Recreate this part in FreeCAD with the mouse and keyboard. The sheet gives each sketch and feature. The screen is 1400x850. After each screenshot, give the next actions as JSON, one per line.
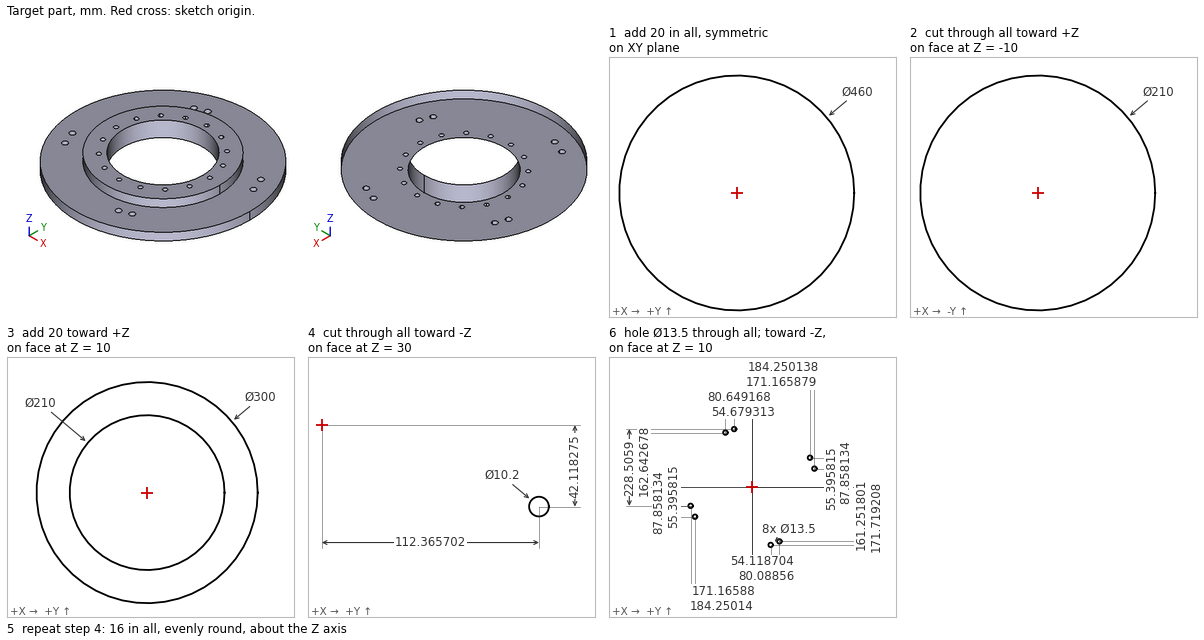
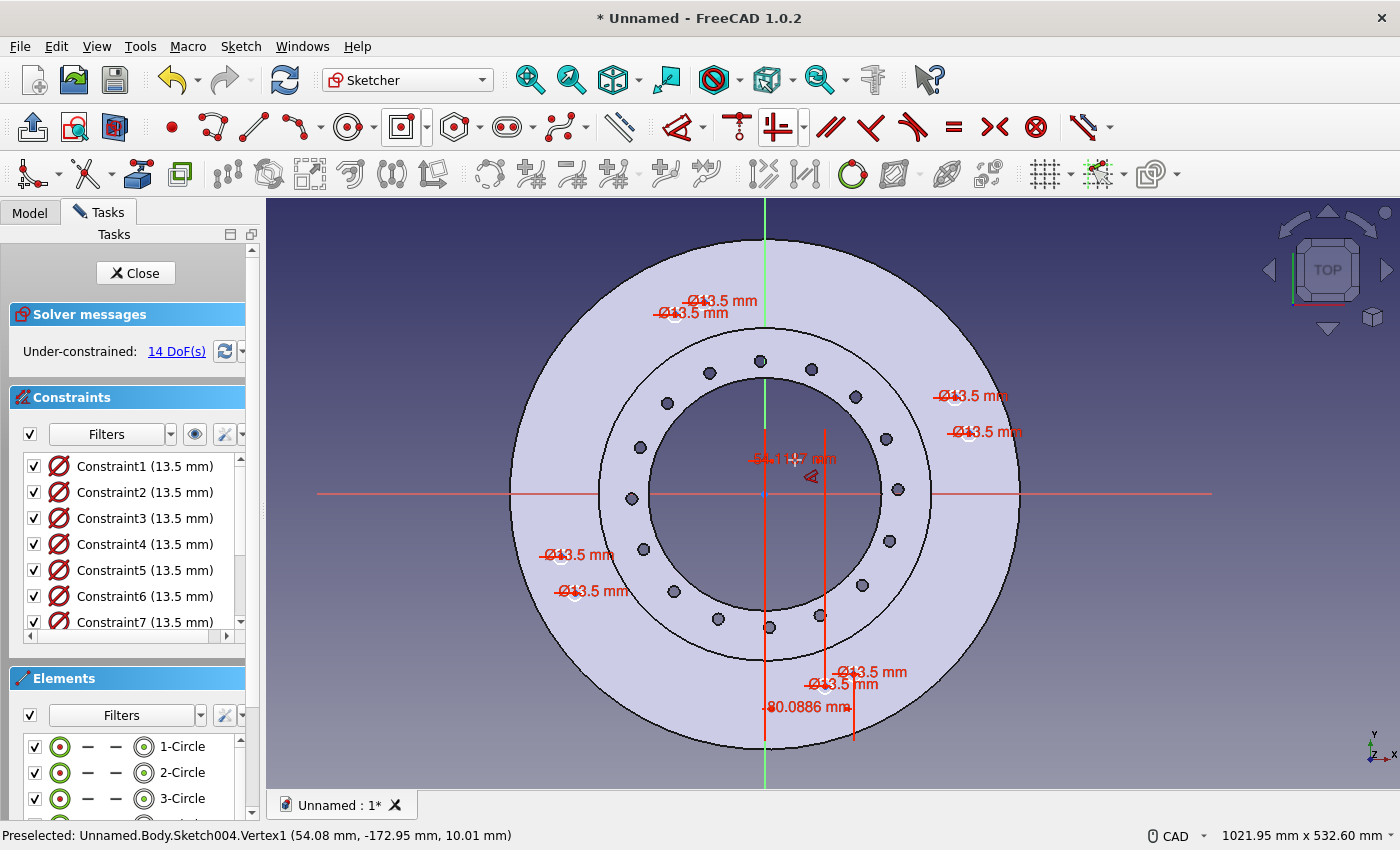
{"action": "left_click", "coordinate": [955, 398]}
{"action": "left_click", "coordinate": [989, 446]}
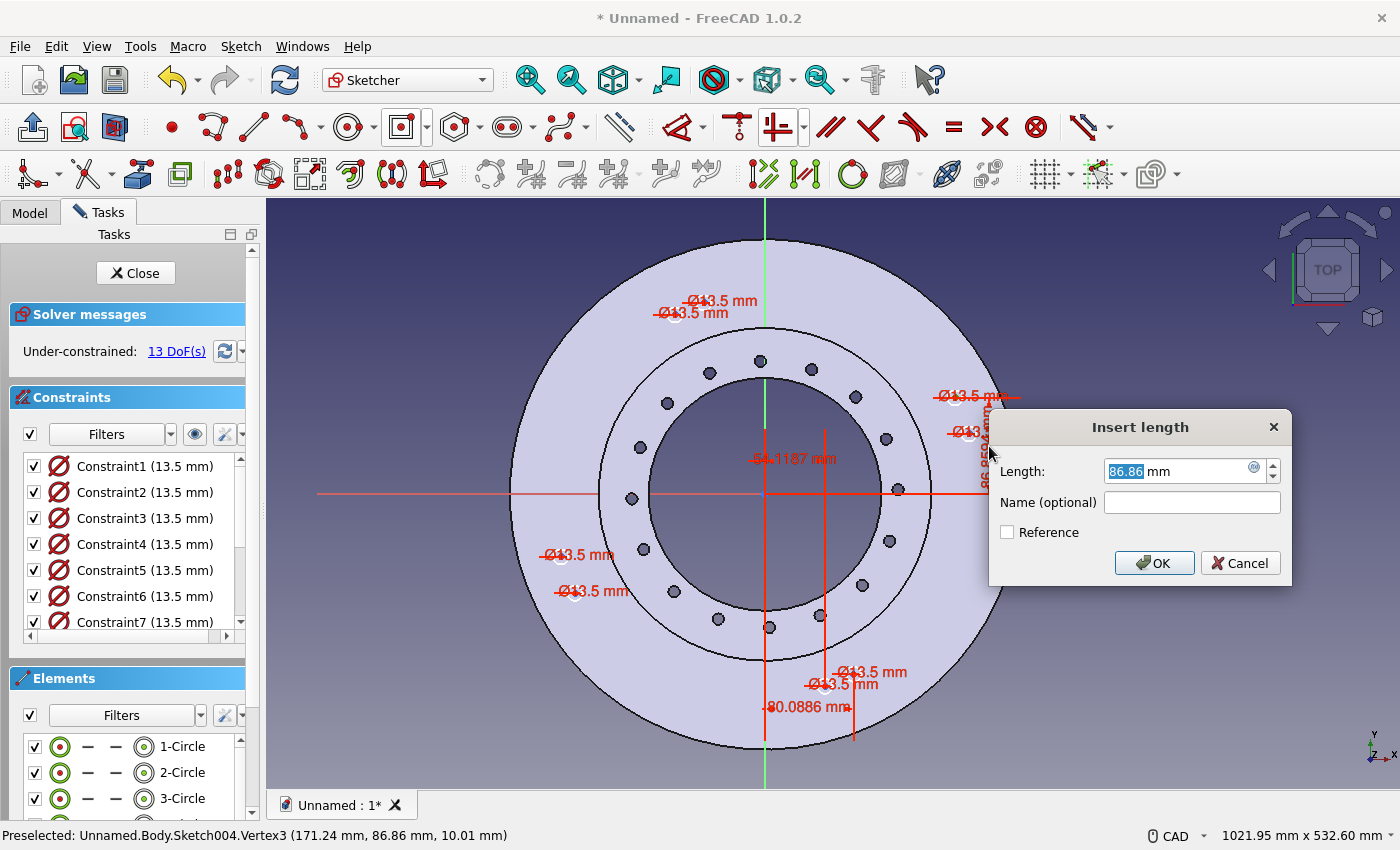
{"action": "type", "text": "87.858134"}
{"action": "key", "text": "Return"}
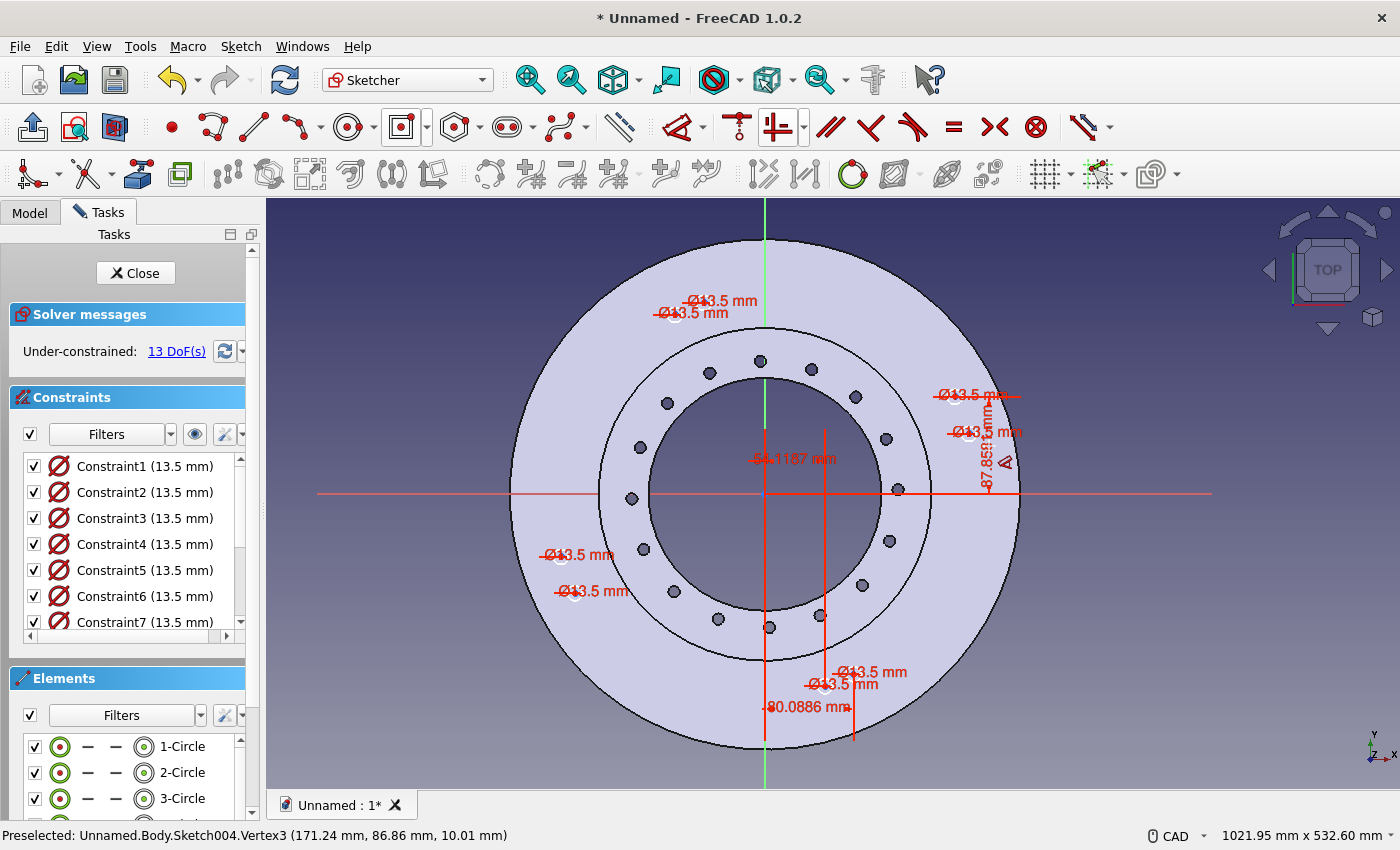
{"action": "left_click", "coordinate": [969, 434]}
{"action": "left_click", "coordinate": [1003, 478]}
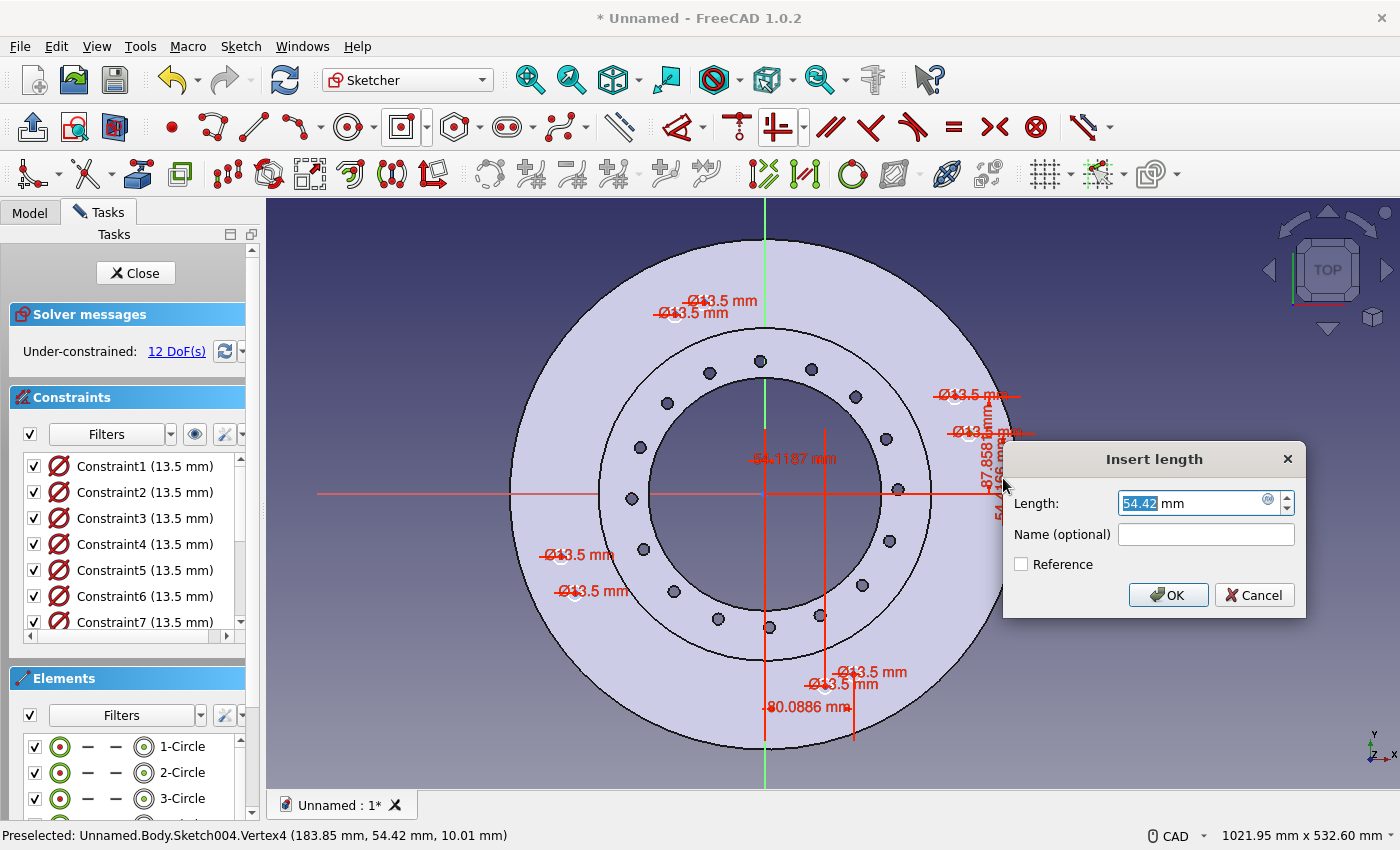
{"action": "type", "text": "55.395815"}
{"action": "key", "text": "Return"}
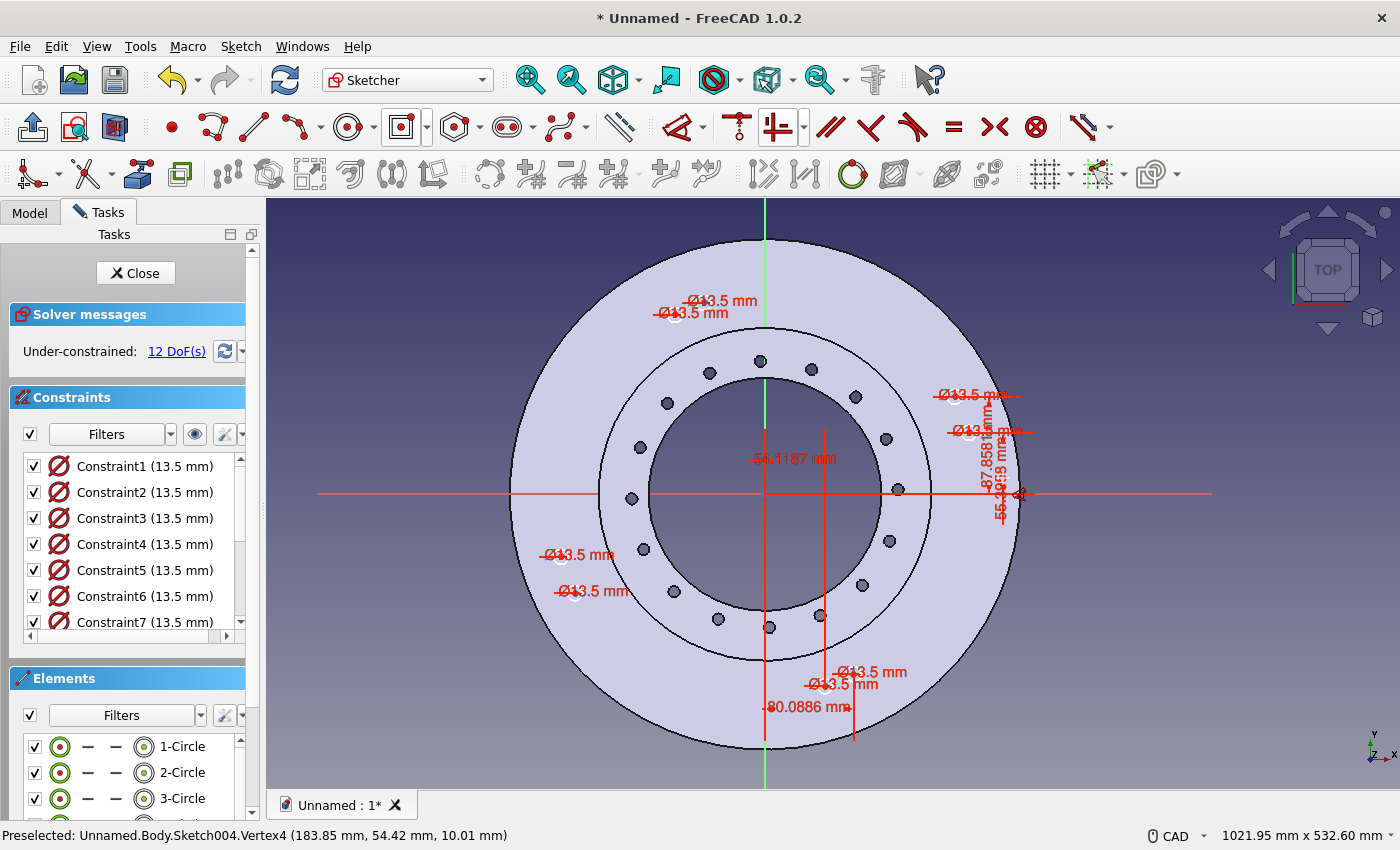
{"action": "left_click", "coordinate": [575, 593]}
{"action": "left_click", "coordinate": [670, 627]}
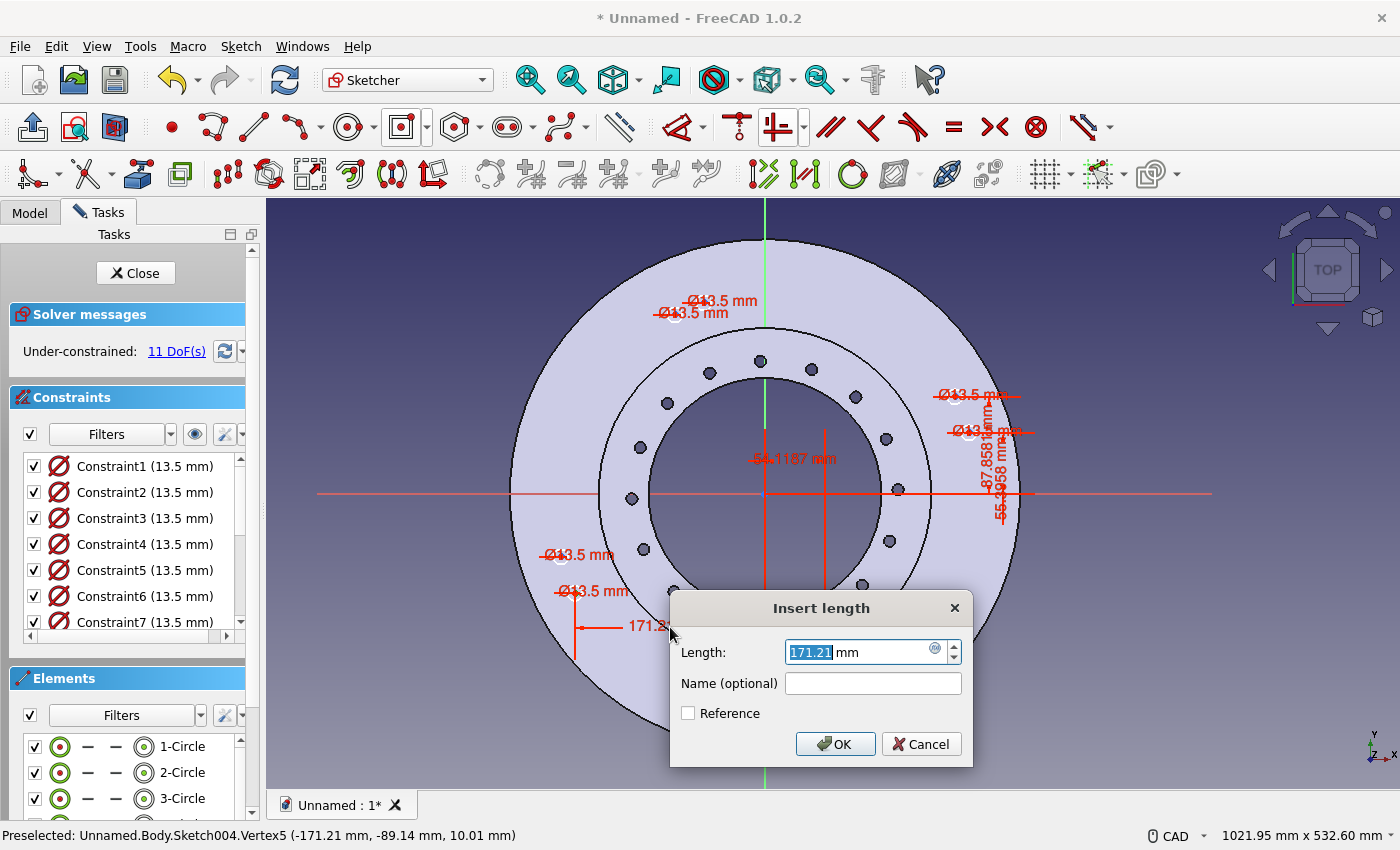
{"action": "type", "text": "171.16588"}
{"action": "key", "text": "Return"}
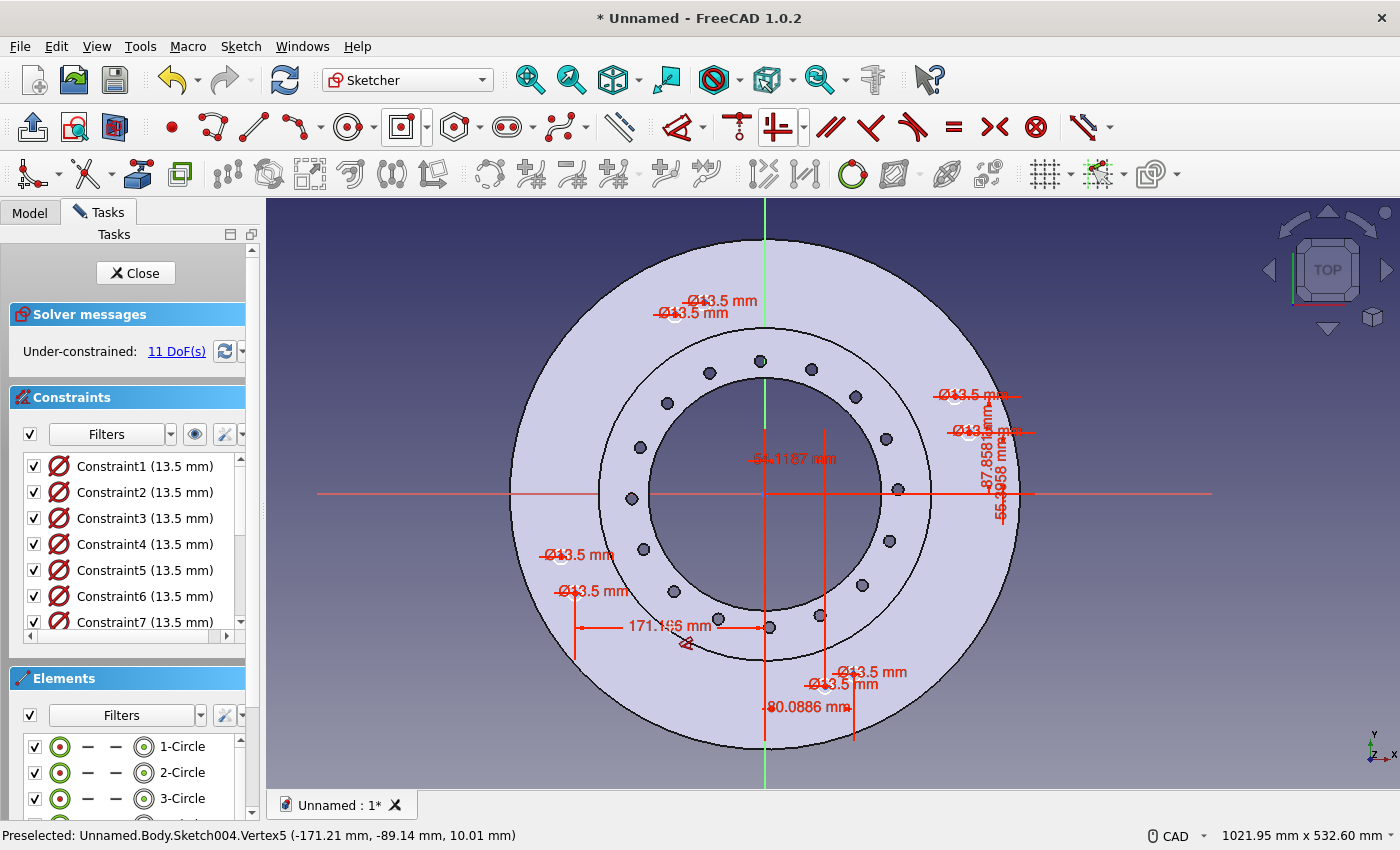
{"action": "left_click", "coordinate": [575, 593]}
{"action": "left_click", "coordinate": [541, 544]}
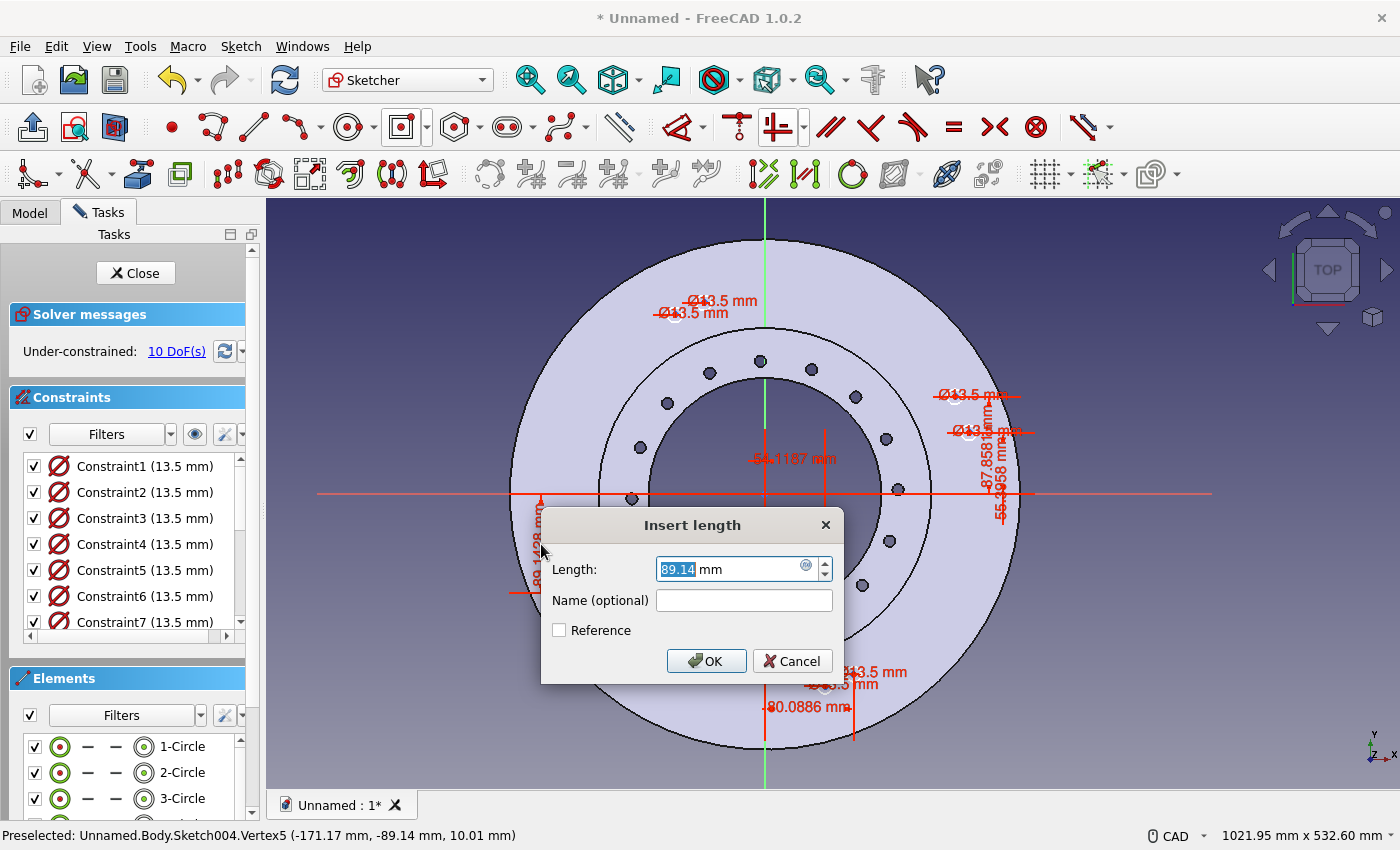
{"action": "type", "text": "87.858134"}
{"action": "key", "text": "Return"}